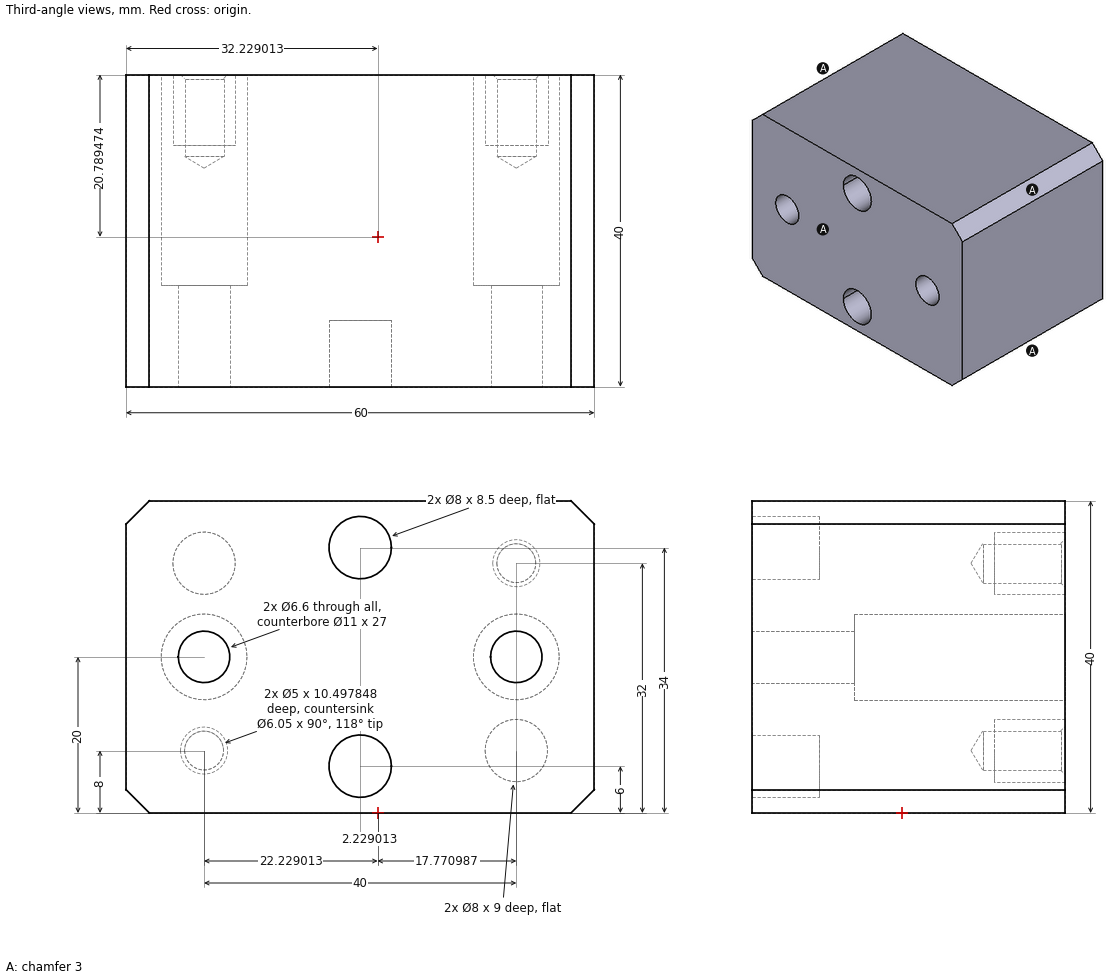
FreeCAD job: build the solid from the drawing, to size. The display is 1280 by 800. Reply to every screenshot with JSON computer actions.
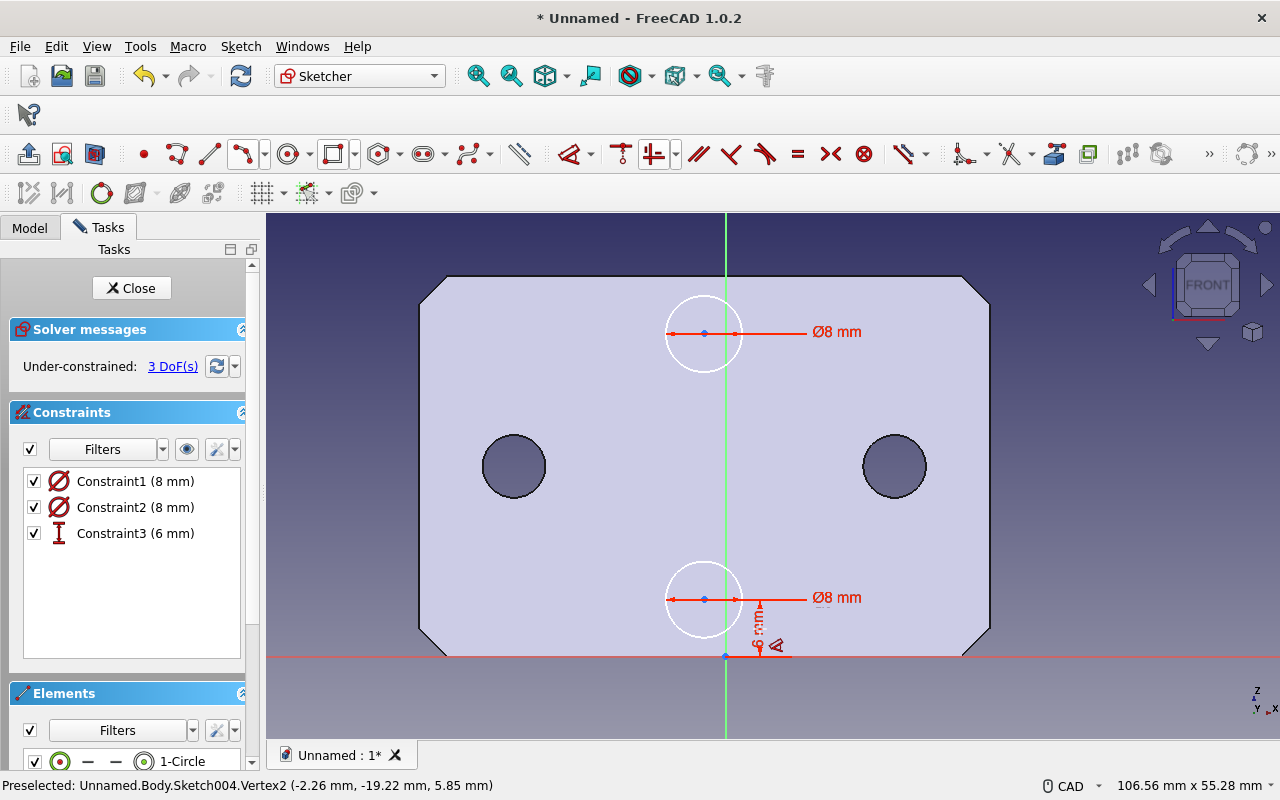
{"action": "left_click", "coordinate": [704, 334]}
{"action": "left_click", "coordinate": [760, 495]}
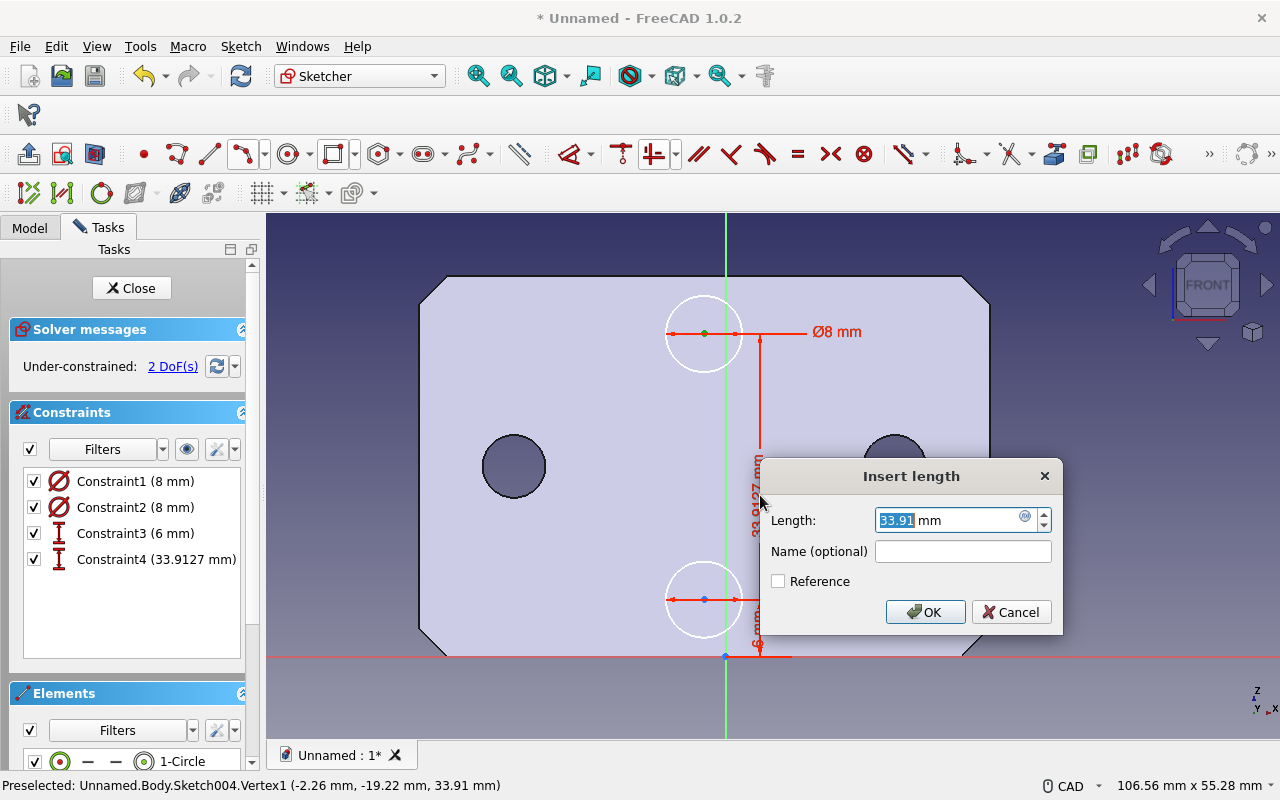
{"action": "type", "text": "34"}
{"action": "key", "text": "Return"}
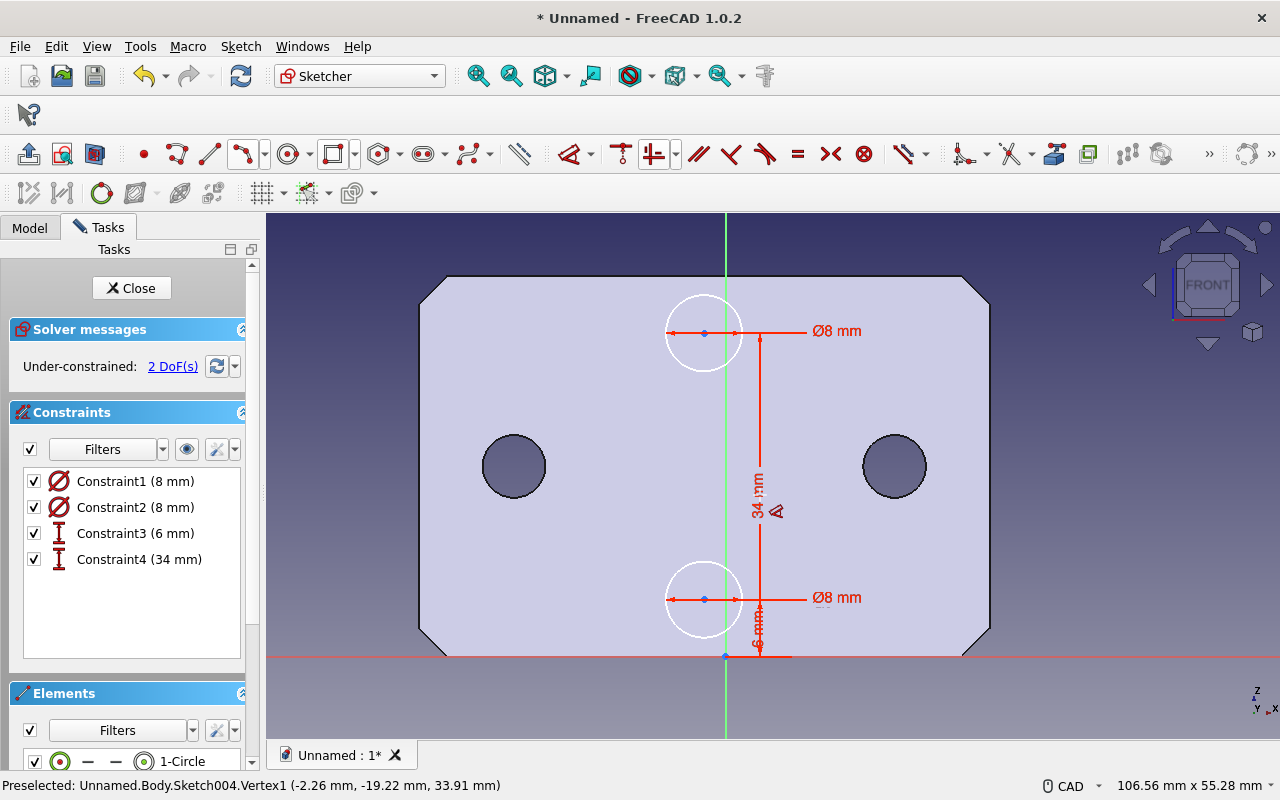
{"action": "scroll", "coordinate": [704, 333], "scroll_direction": "up", "scroll_amount": 4}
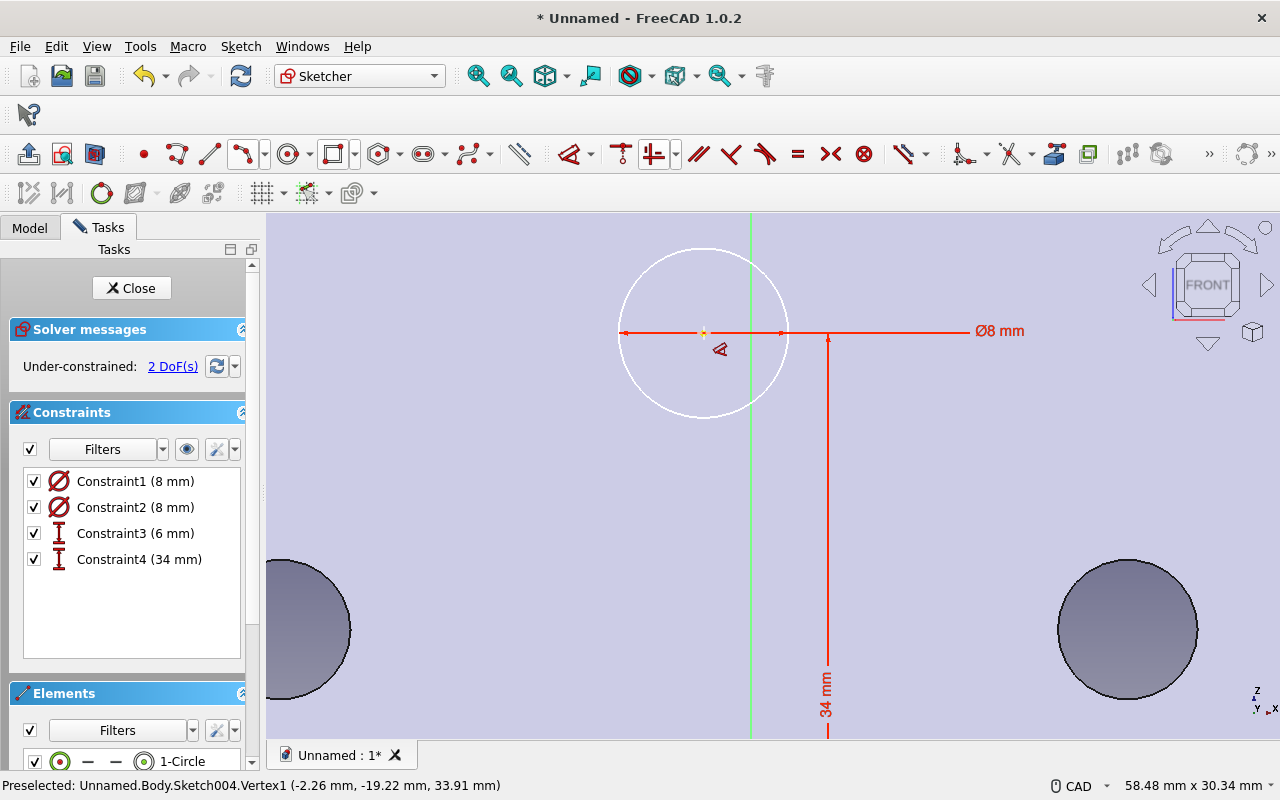
{"action": "left_click", "coordinate": [703, 333]}
{"action": "left_click", "coordinate": [727, 299]}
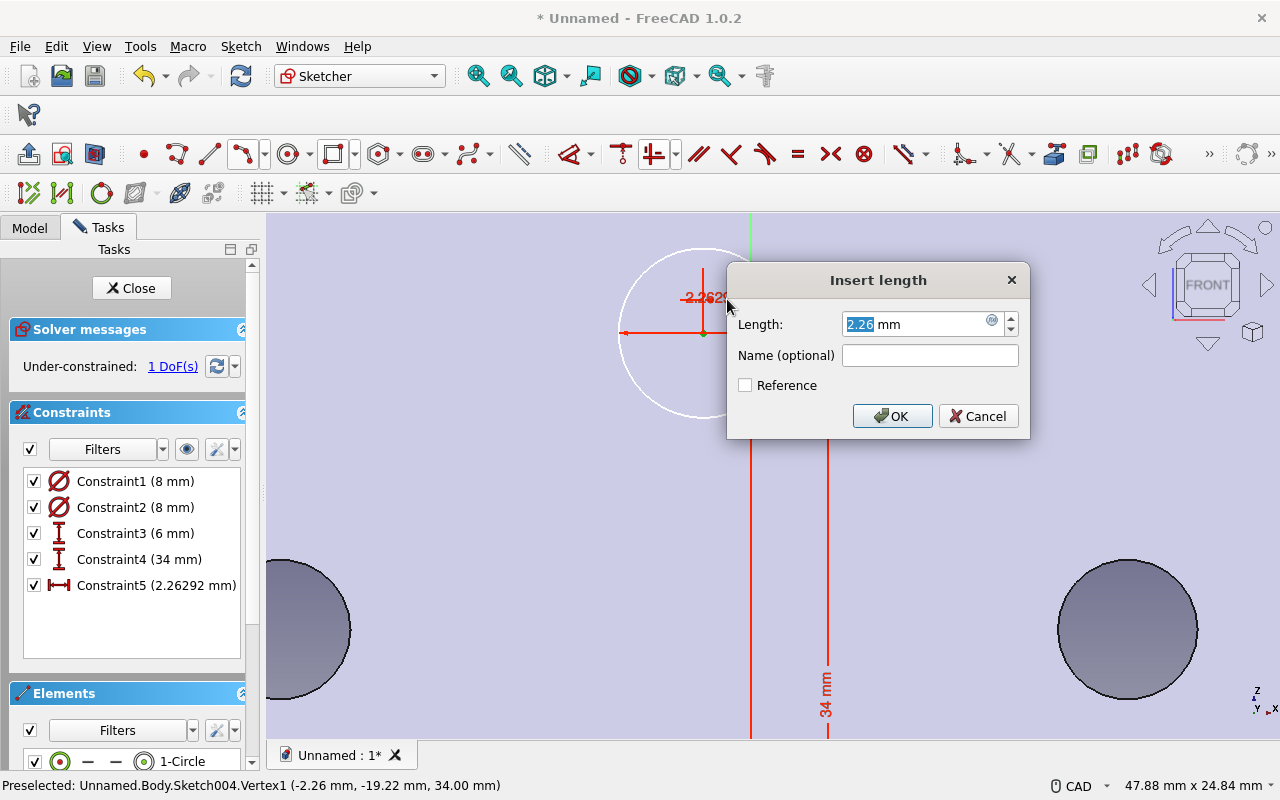
{"action": "type", "text": "2.229013"}
{"action": "key", "text": "Return"}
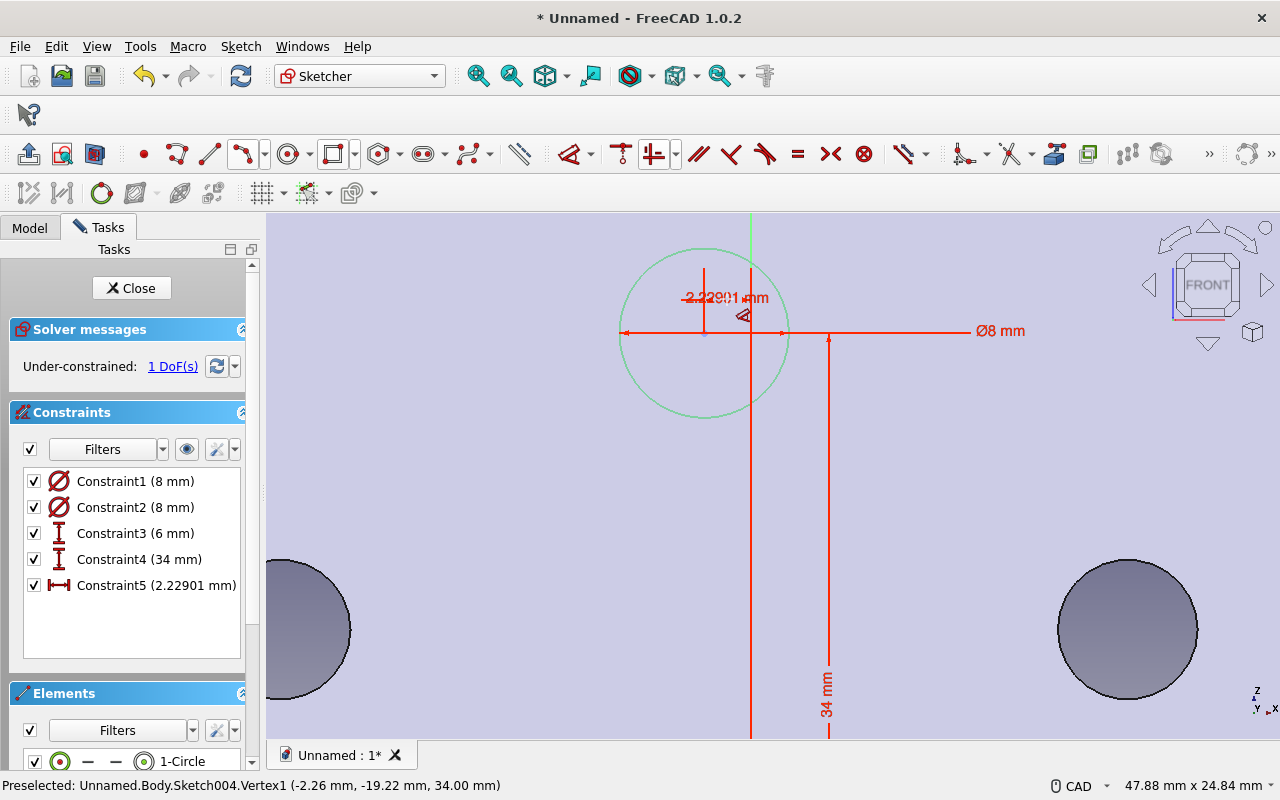
{"action": "scroll", "coordinate": [705, 333], "scroll_direction": "down", "scroll_amount": 4}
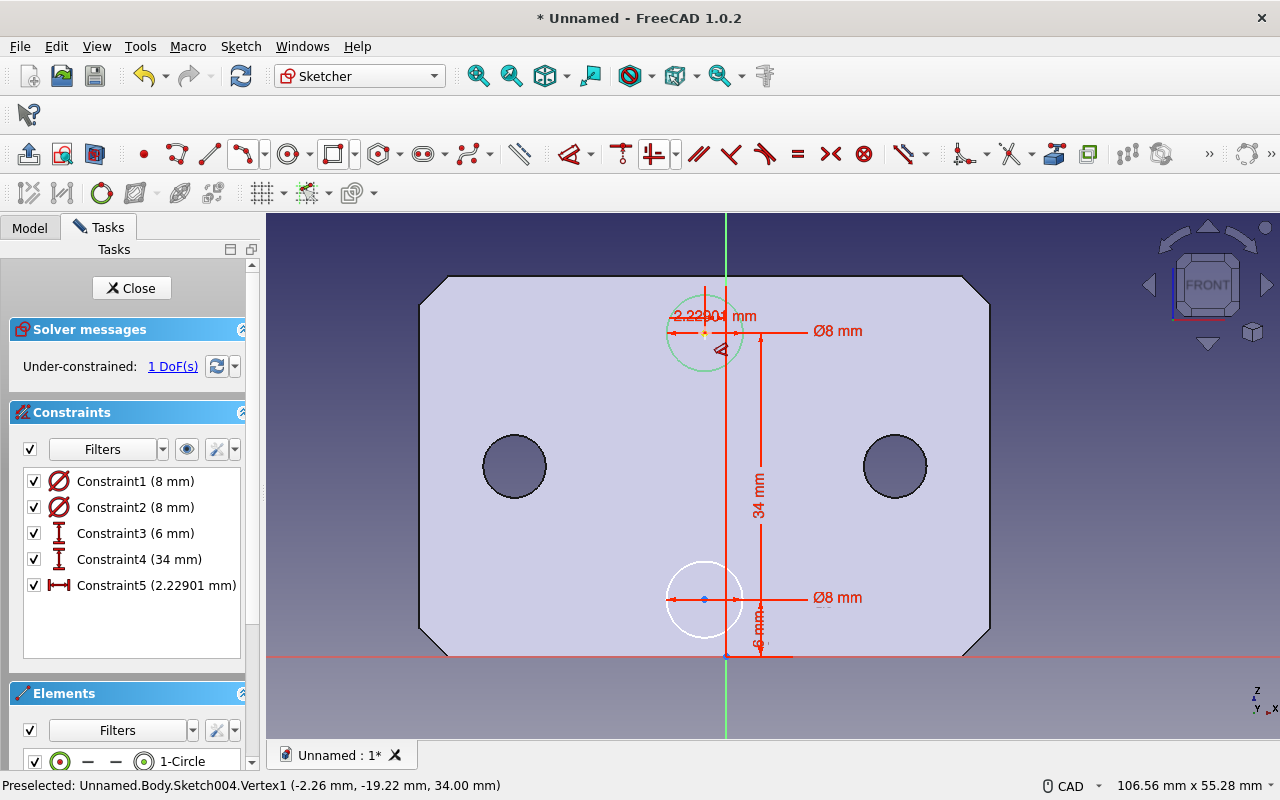
{"action": "scroll", "coordinate": [705, 600], "scroll_direction": "up", "scroll_amount": 4}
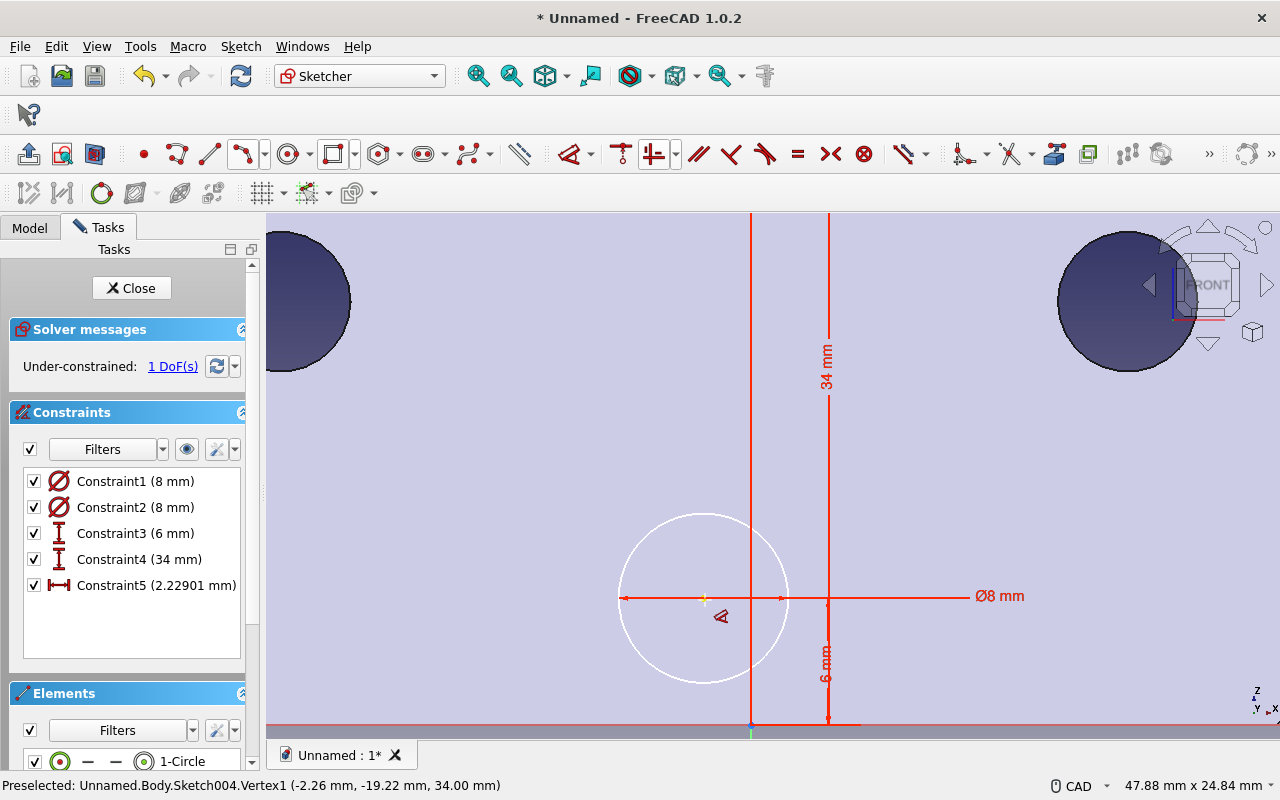
{"action": "left_click", "coordinate": [703, 598]}
{"action": "left_click", "coordinate": [727, 564]}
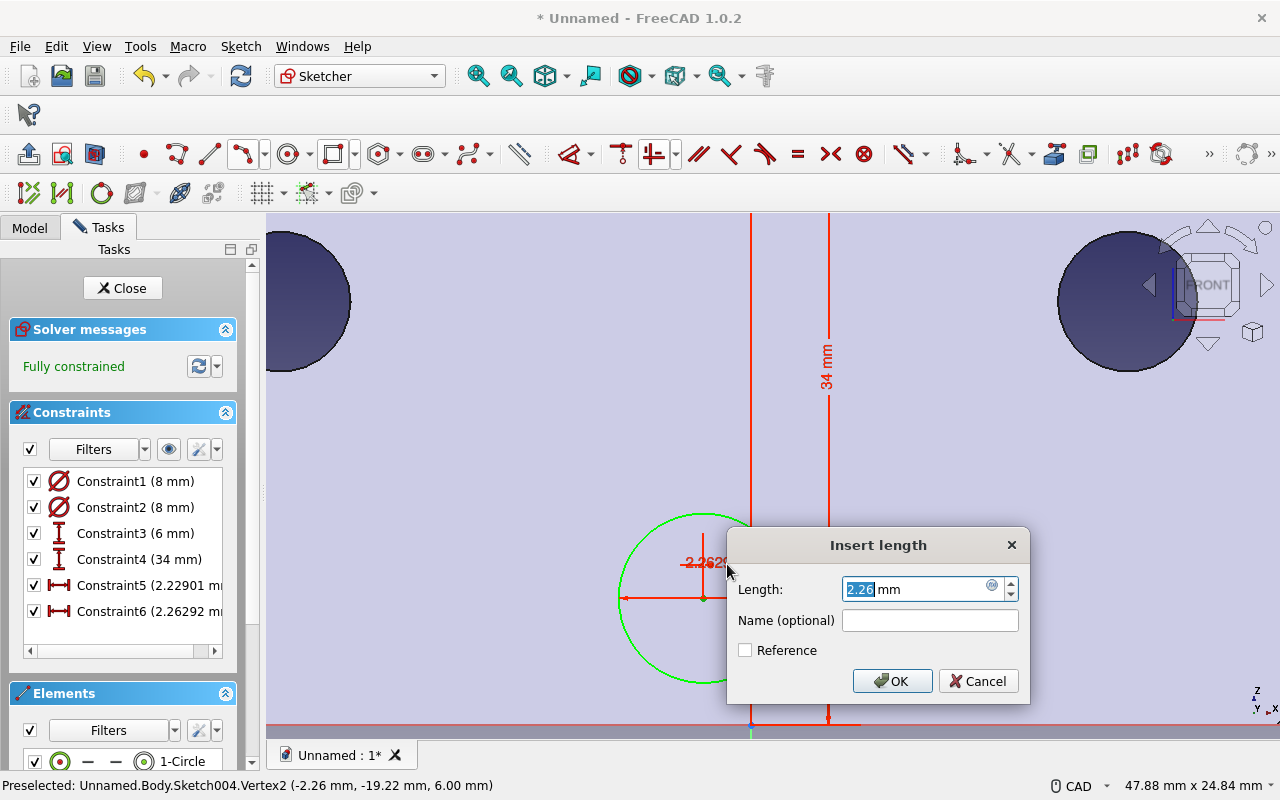
{"action": "type", "text": "2.229013"}
{"action": "key", "text": "Return"}
{"action": "key", "text": "Escape"}